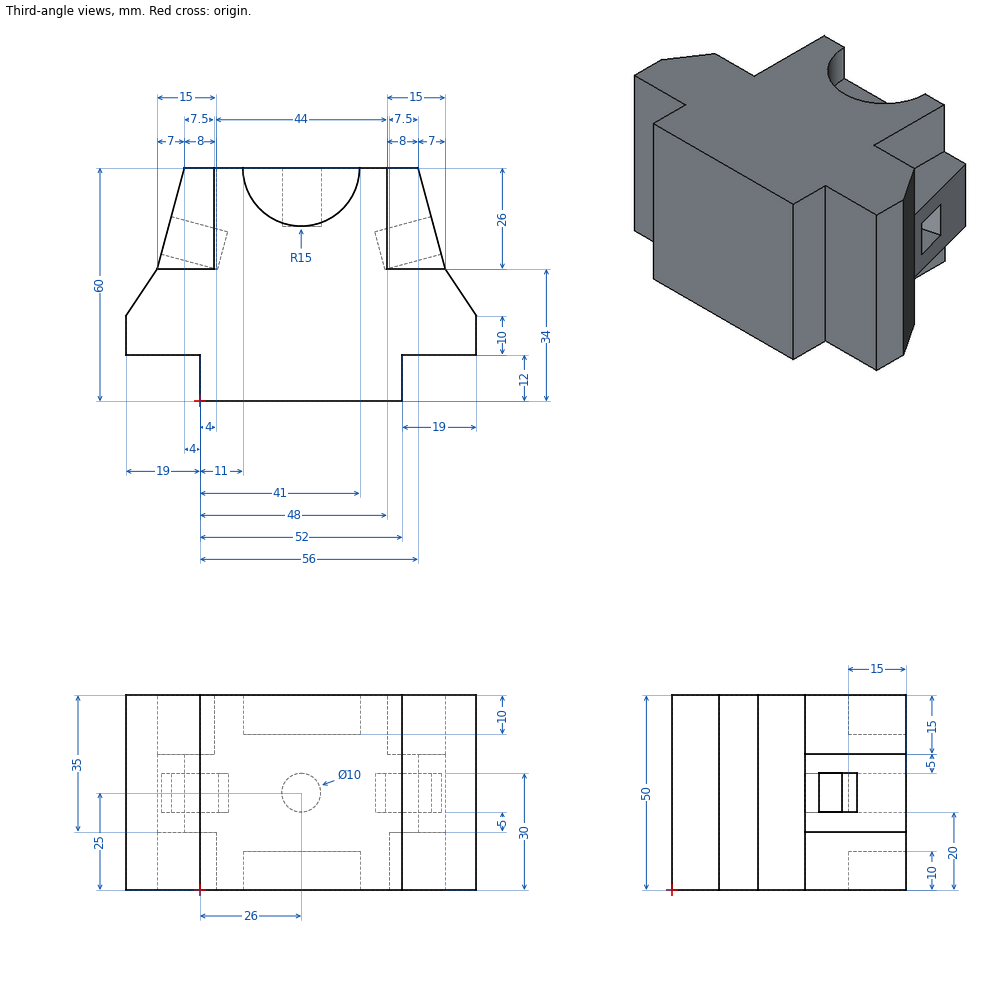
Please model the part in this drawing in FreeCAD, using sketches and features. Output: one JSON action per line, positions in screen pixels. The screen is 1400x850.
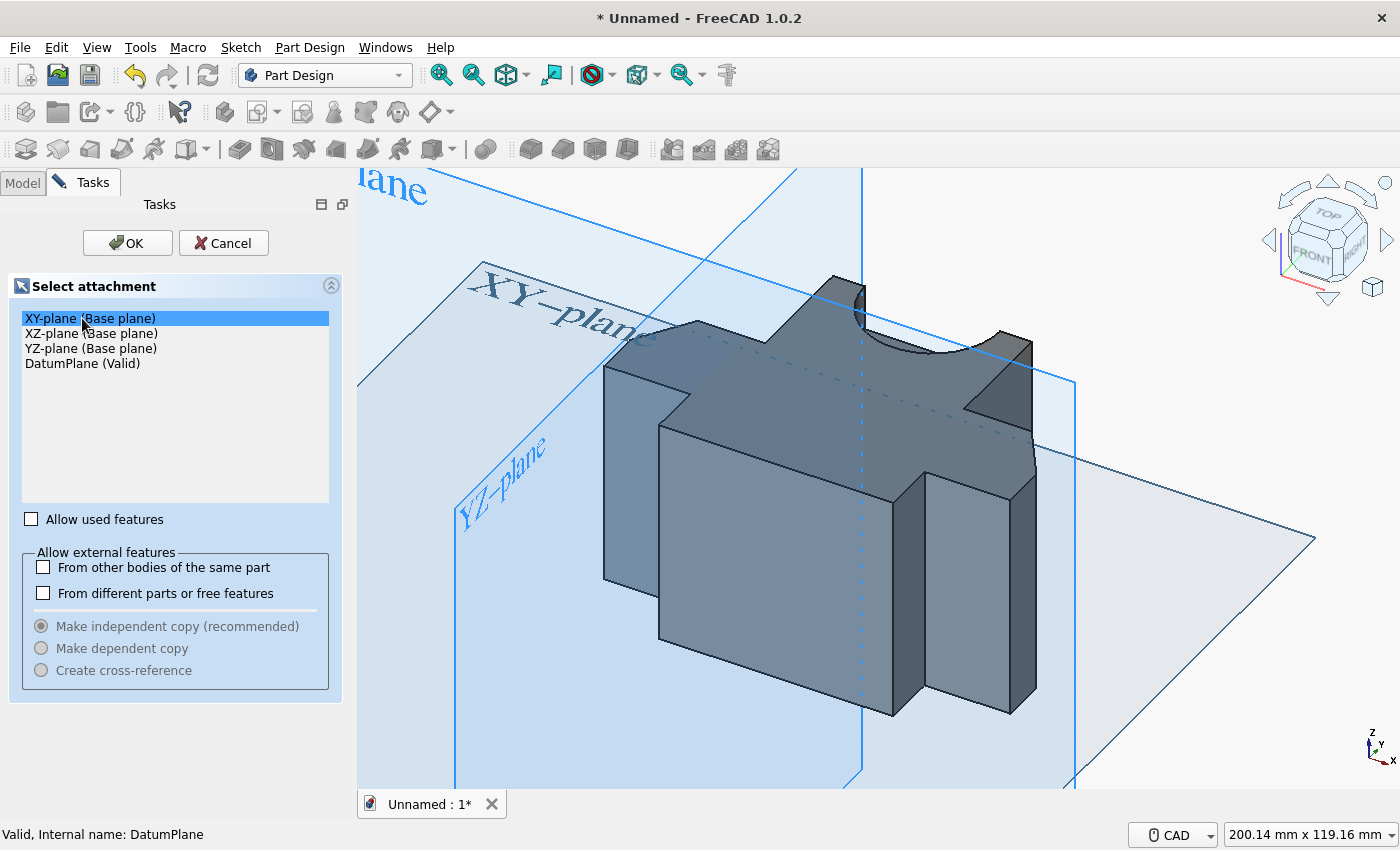
{"action": "left_click", "coordinate": [128, 243]}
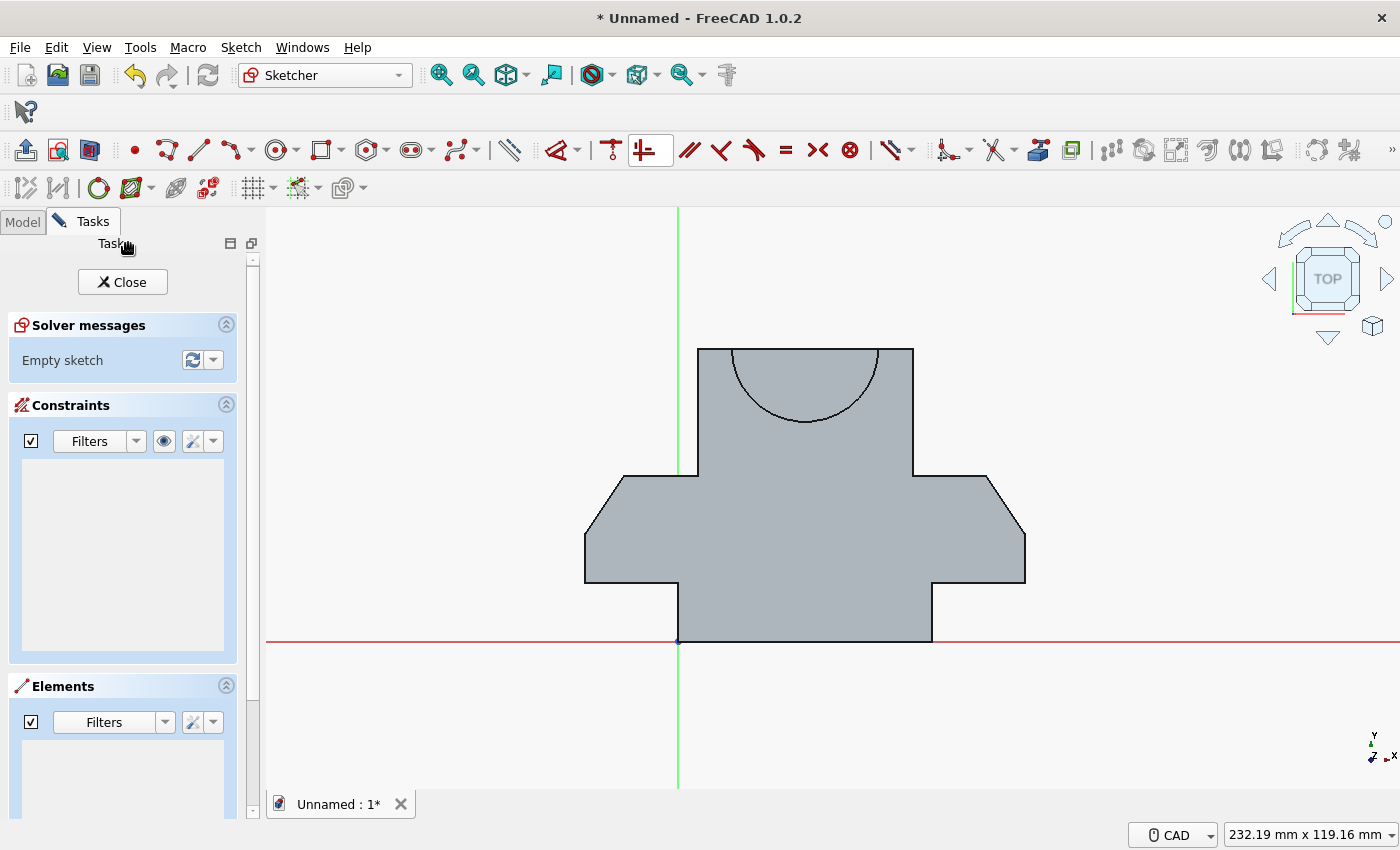
{"action": "left_click", "coordinate": [90, 150]}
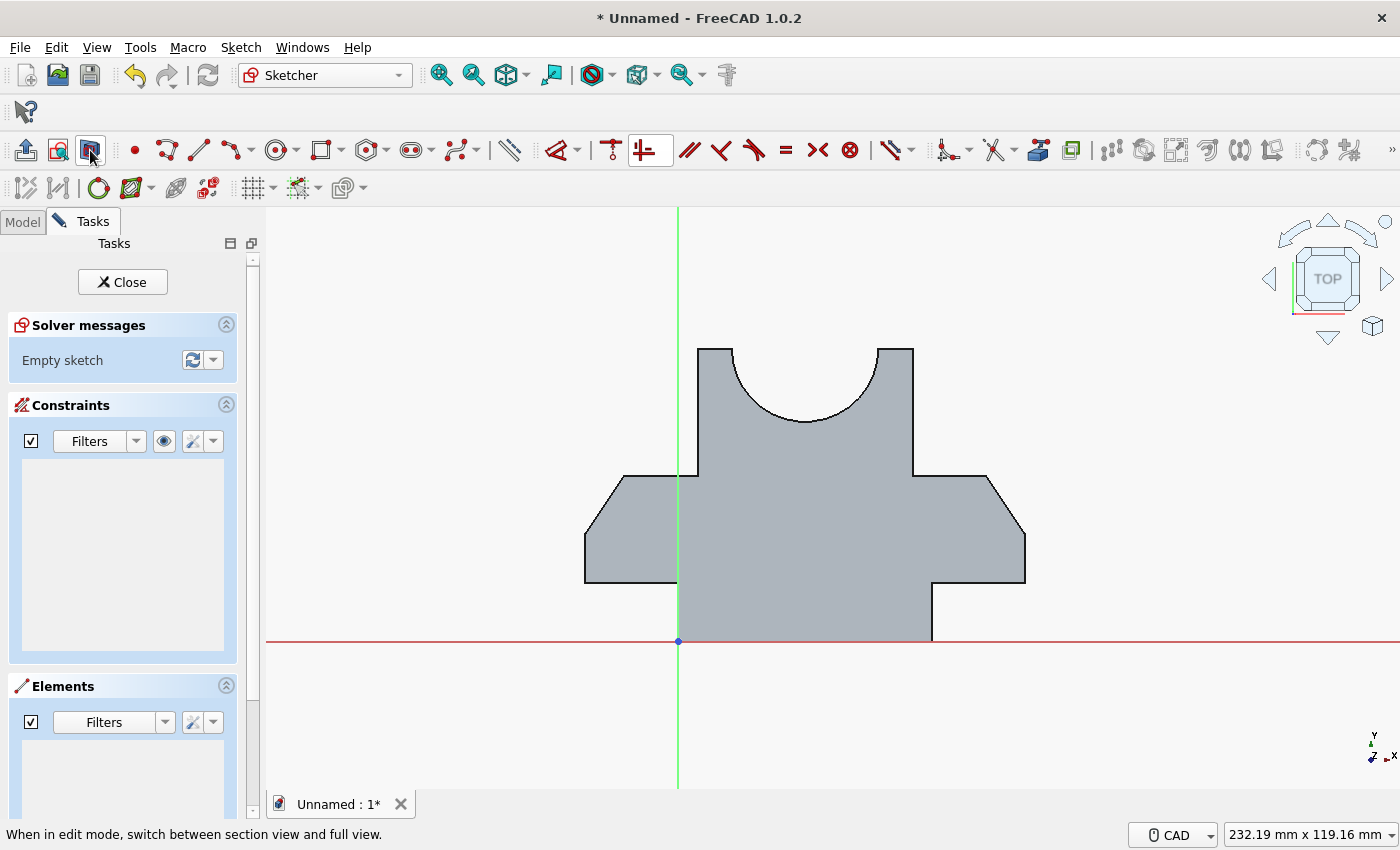
{"action": "left_click", "coordinate": [168, 150]}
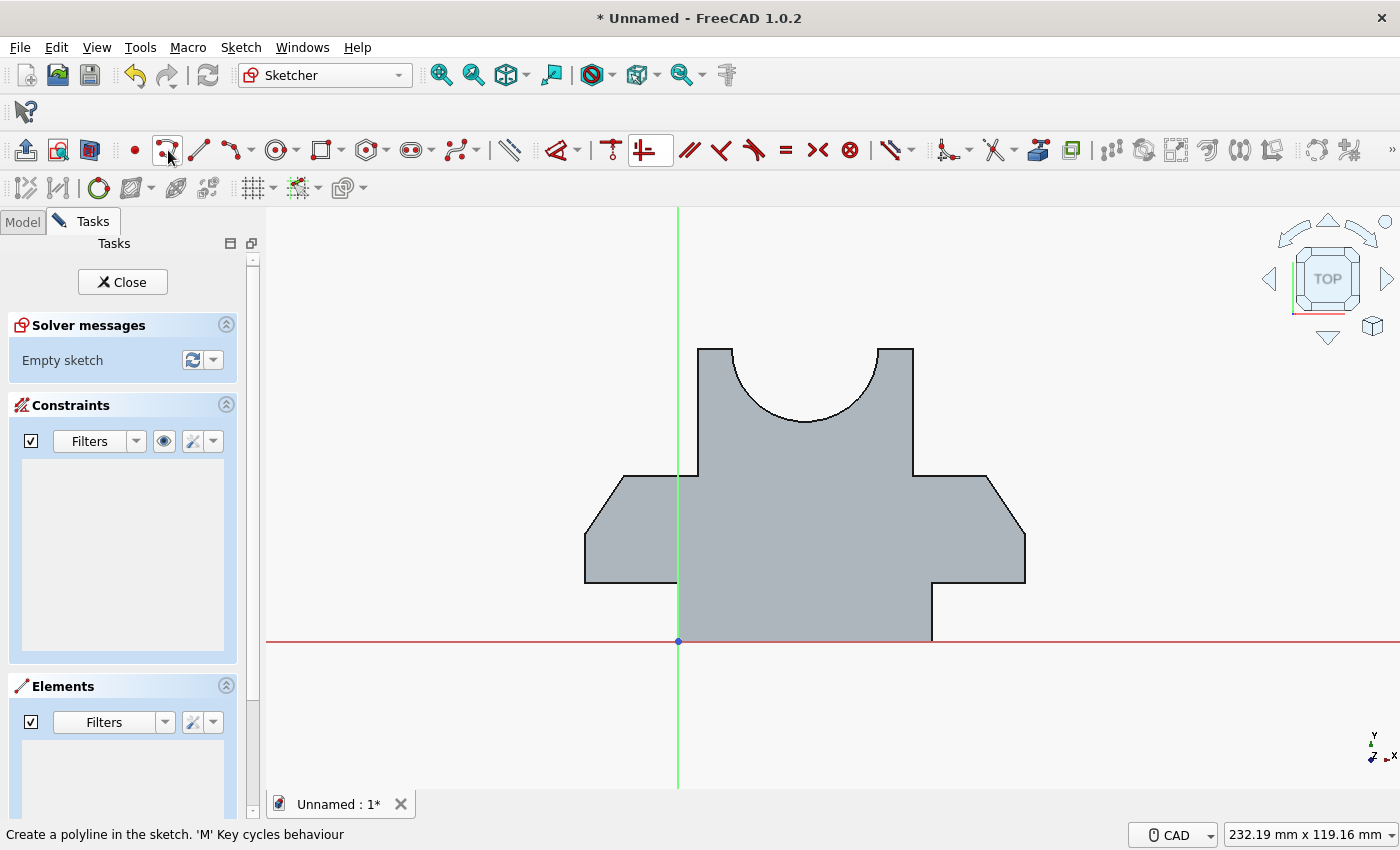
{"action": "left_click", "coordinate": [913, 476]}
{"action": "left_click", "coordinate": [913, 349]}
{"action": "left_click", "coordinate": [952, 349]}
{"action": "left_click", "coordinate": [986, 476]}
{"action": "left_click", "coordinate": [913, 477]}
{"action": "key", "text": "Escape"}
{"action": "key", "text": "Escape"}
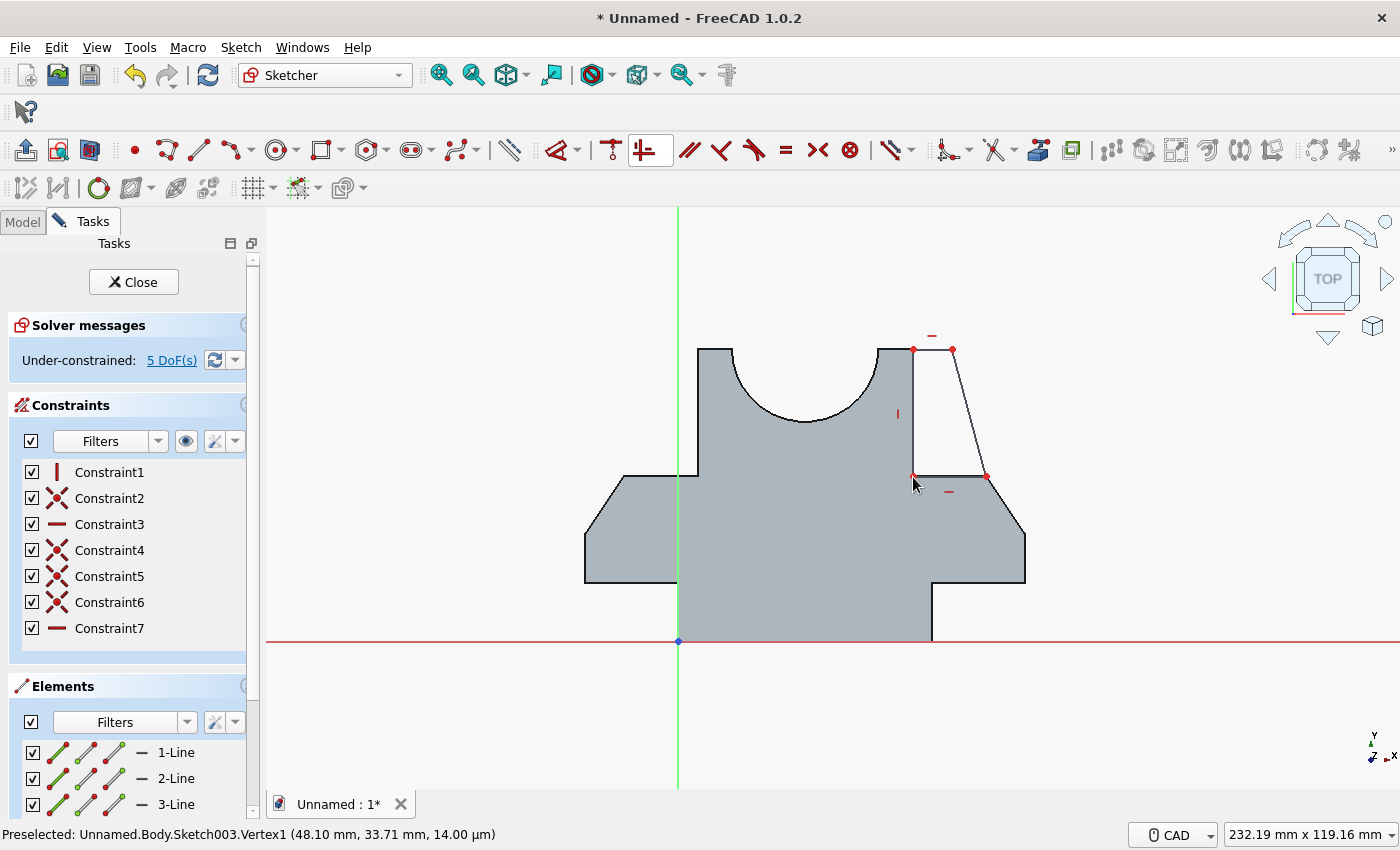
{"action": "left_click", "coordinate": [556, 150]}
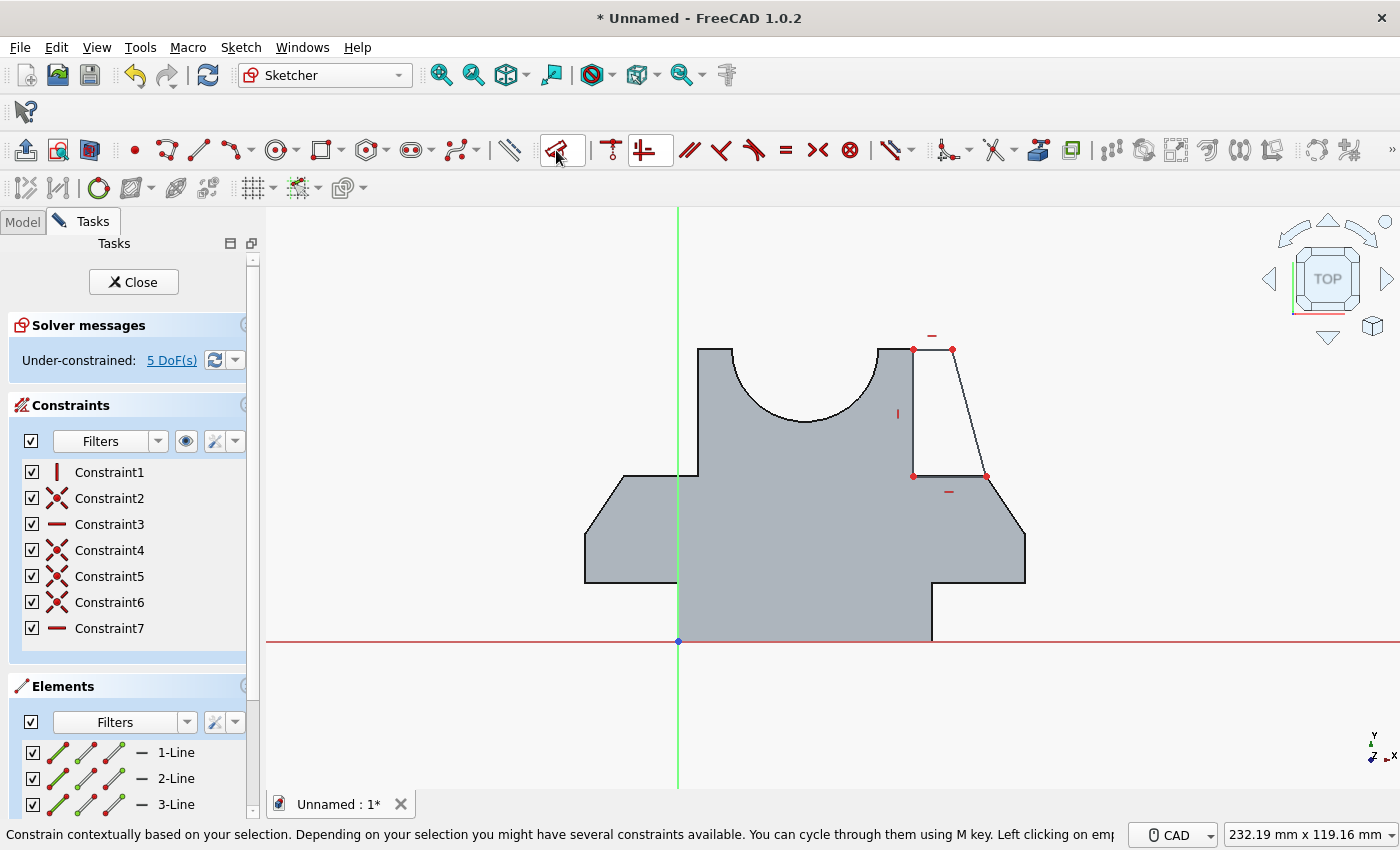
{"action": "left_click", "coordinate": [925, 350]}
{"action": "left_click", "coordinate": [933, 316]}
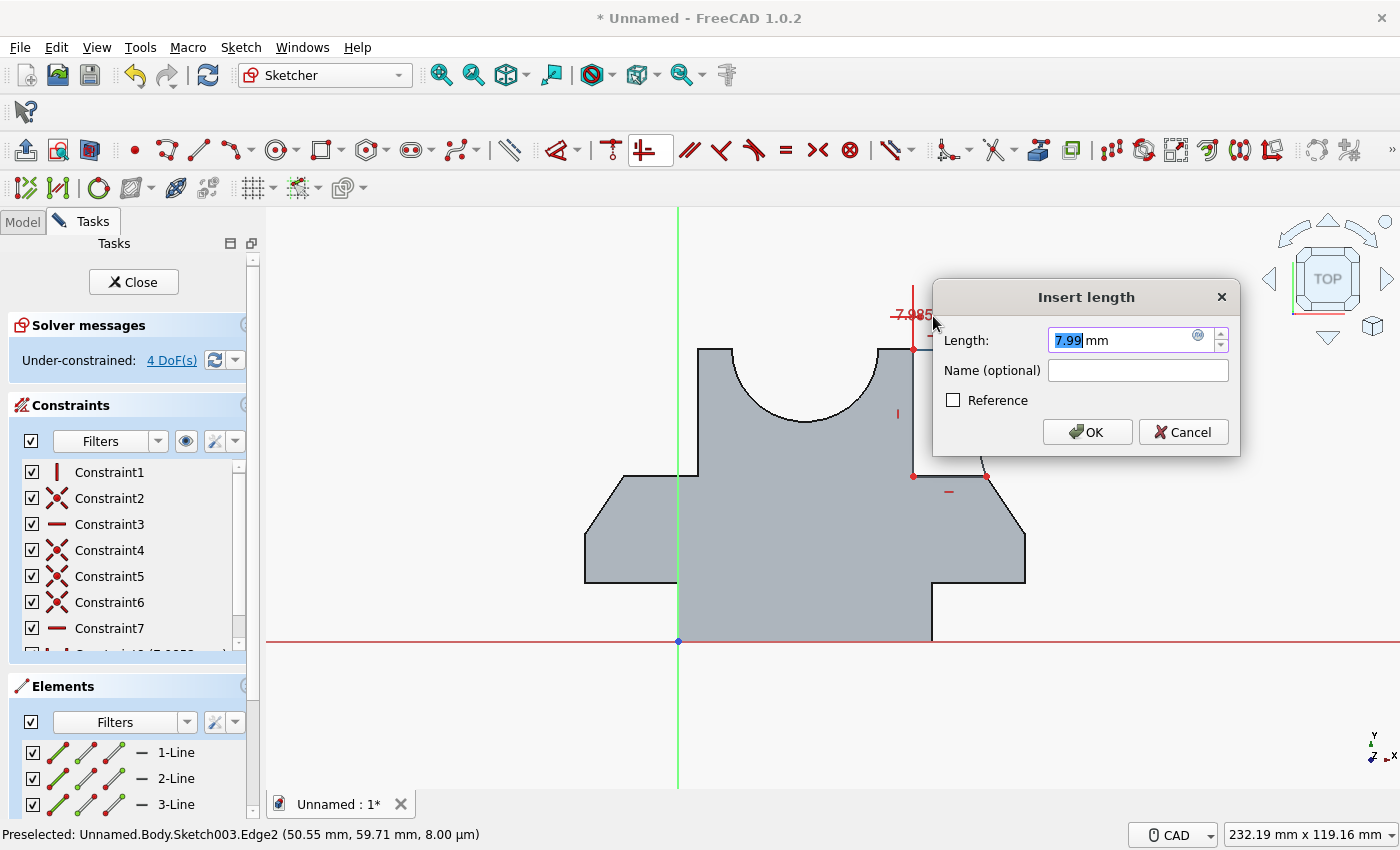
{"action": "type", "text": "8"}
{"action": "key", "text": "Return"}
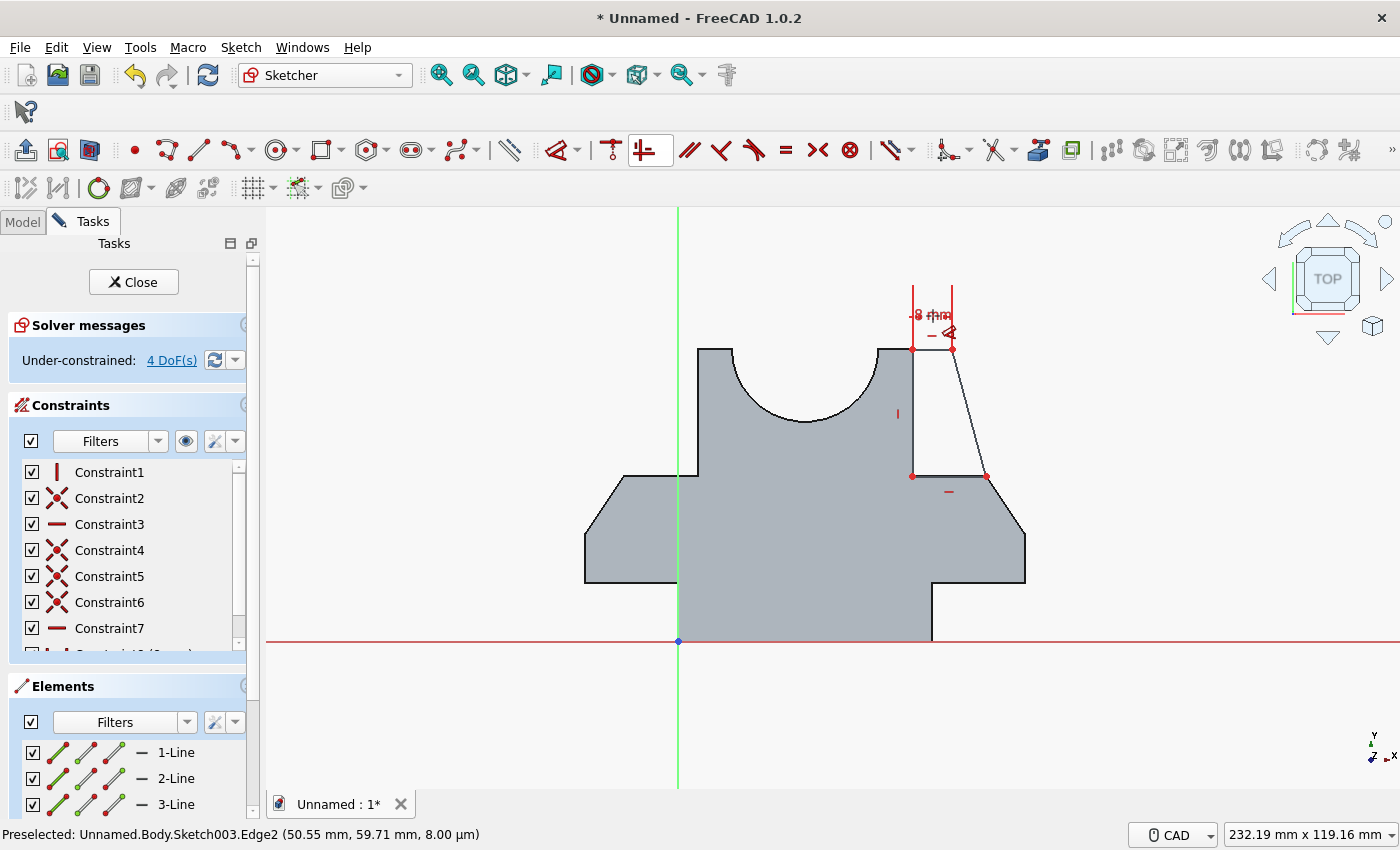
{"action": "left_click", "coordinate": [913, 439]}
{"action": "left_click", "coordinate": [947, 414]}